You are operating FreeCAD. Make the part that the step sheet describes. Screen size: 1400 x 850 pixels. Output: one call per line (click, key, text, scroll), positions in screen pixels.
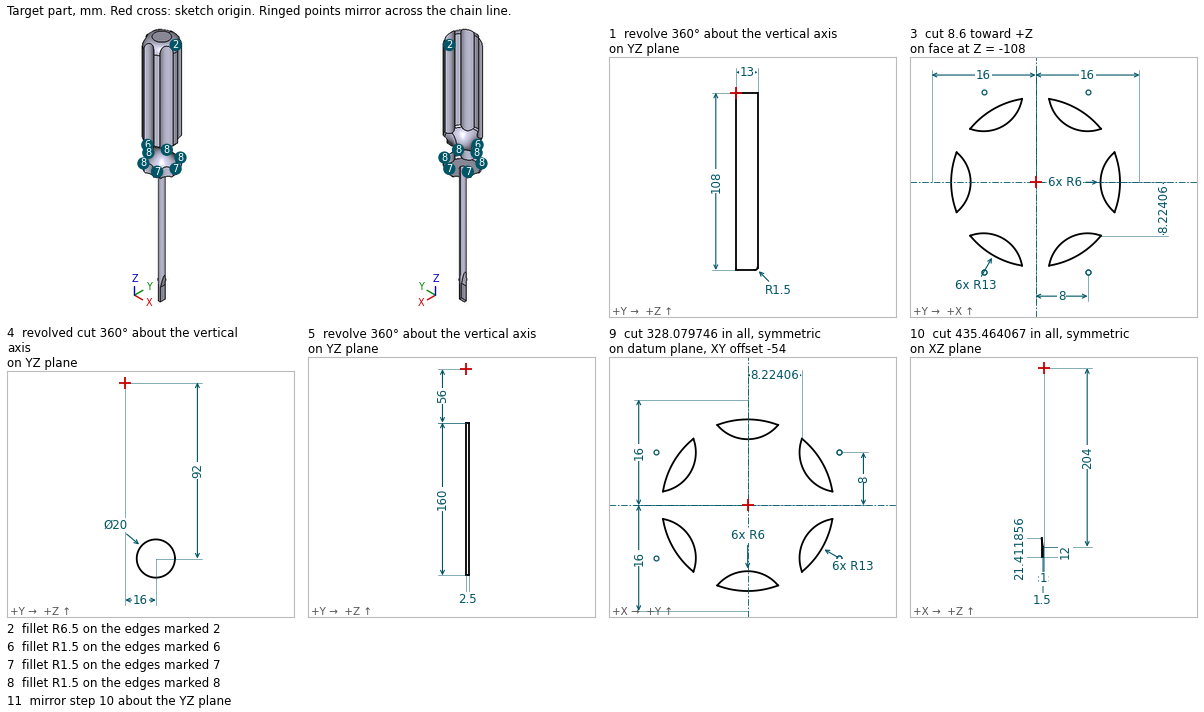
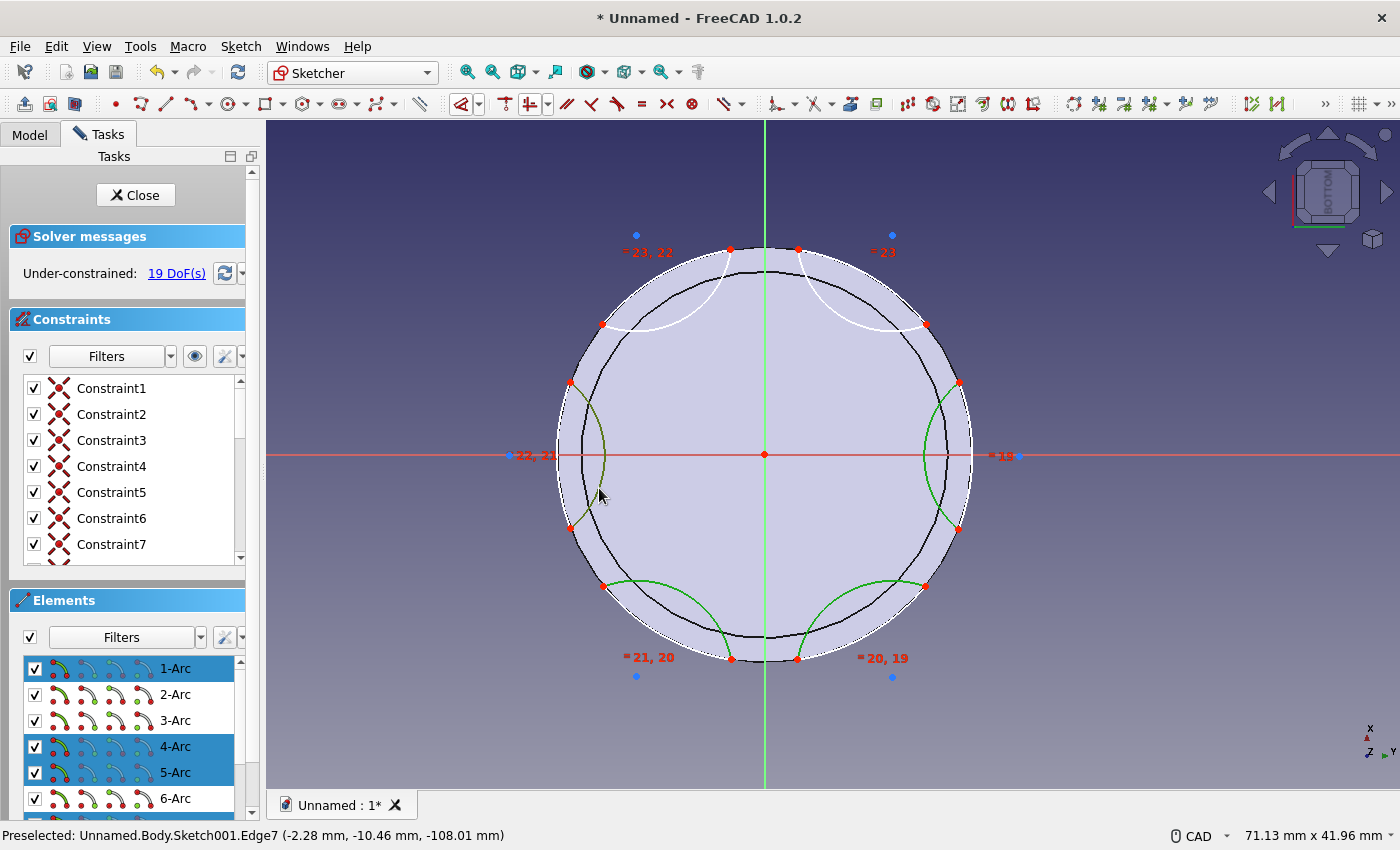
click(653, 330)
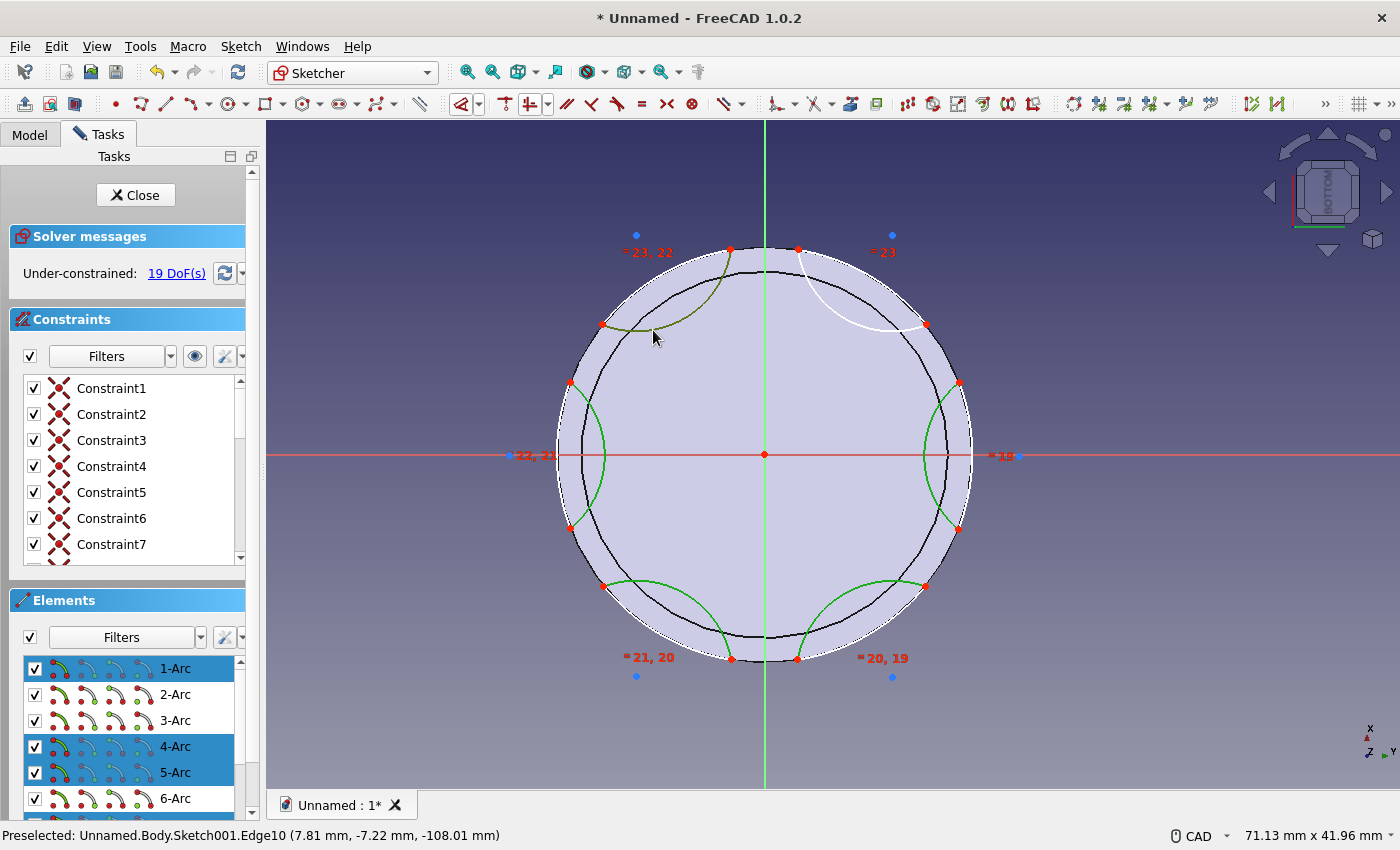
click(818, 296)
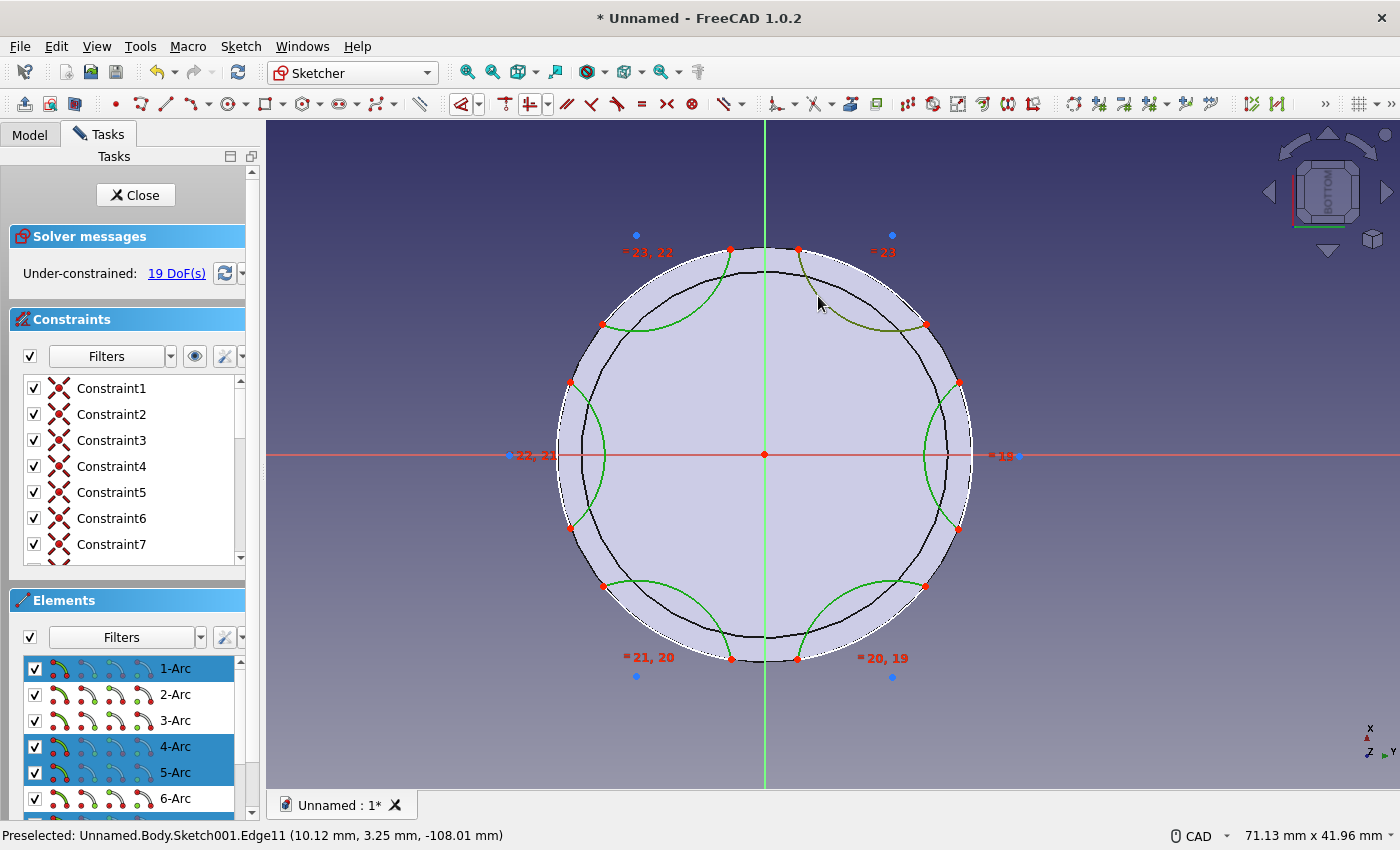
click(642, 104)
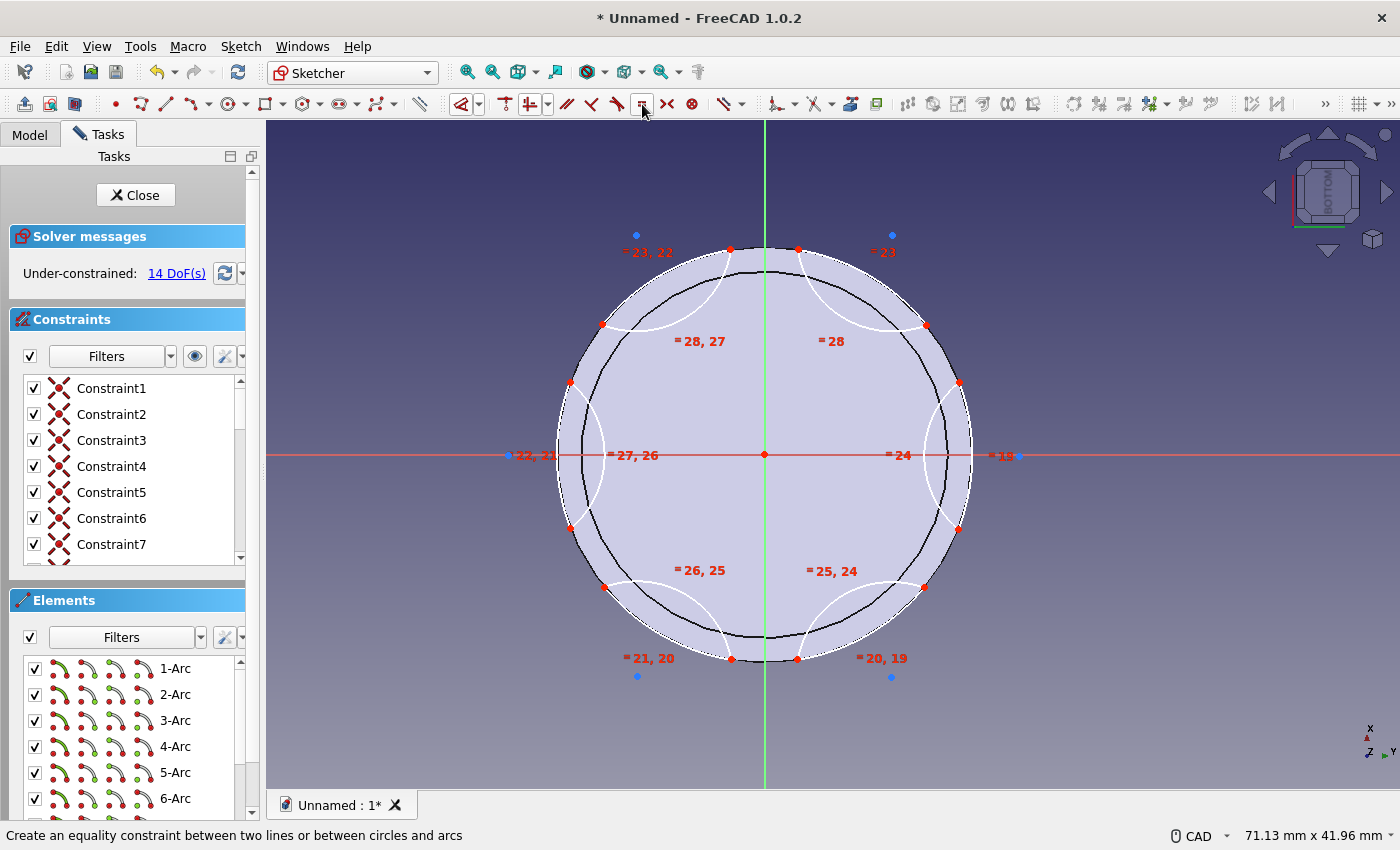
click(1020, 456)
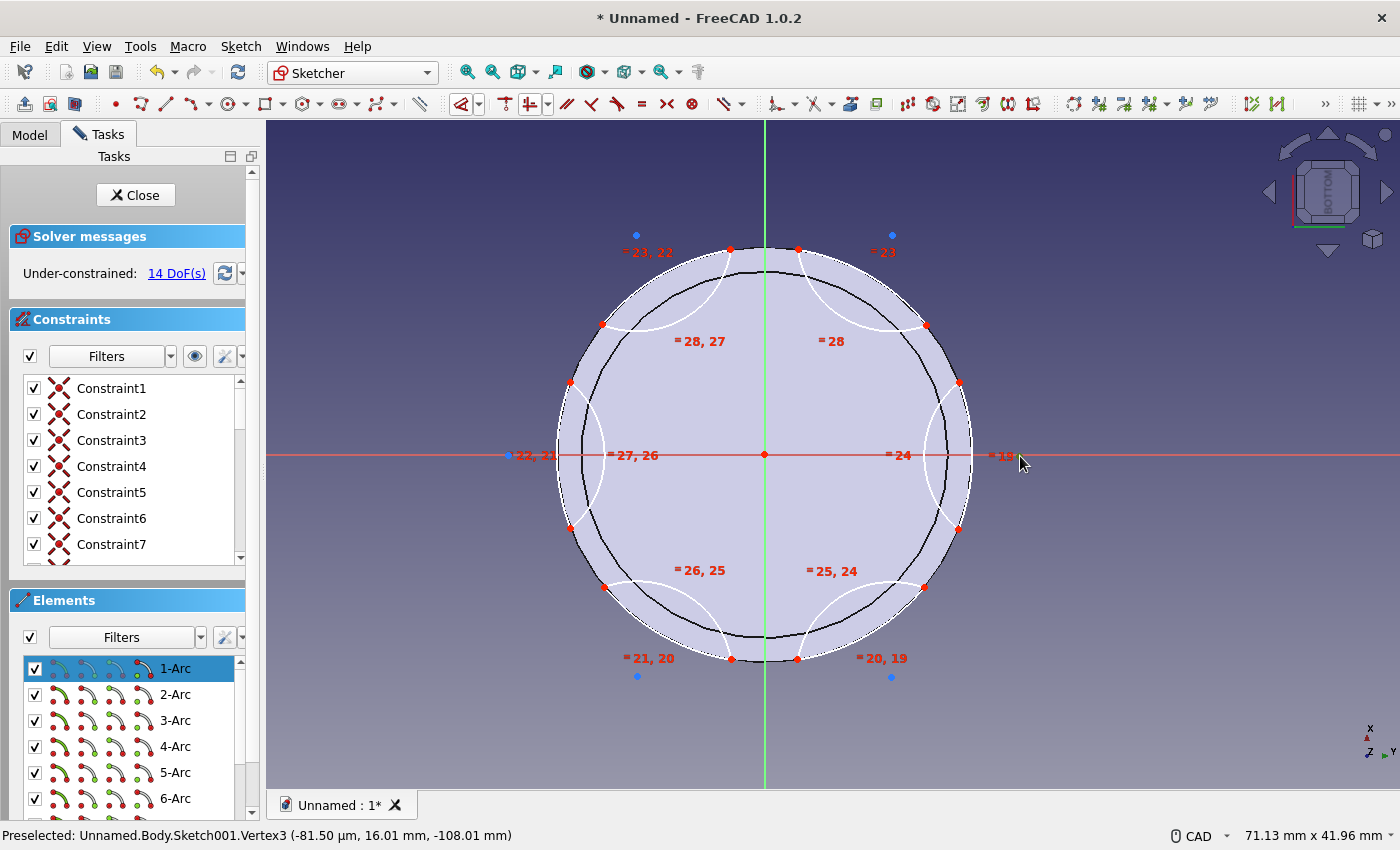
click(361, 455)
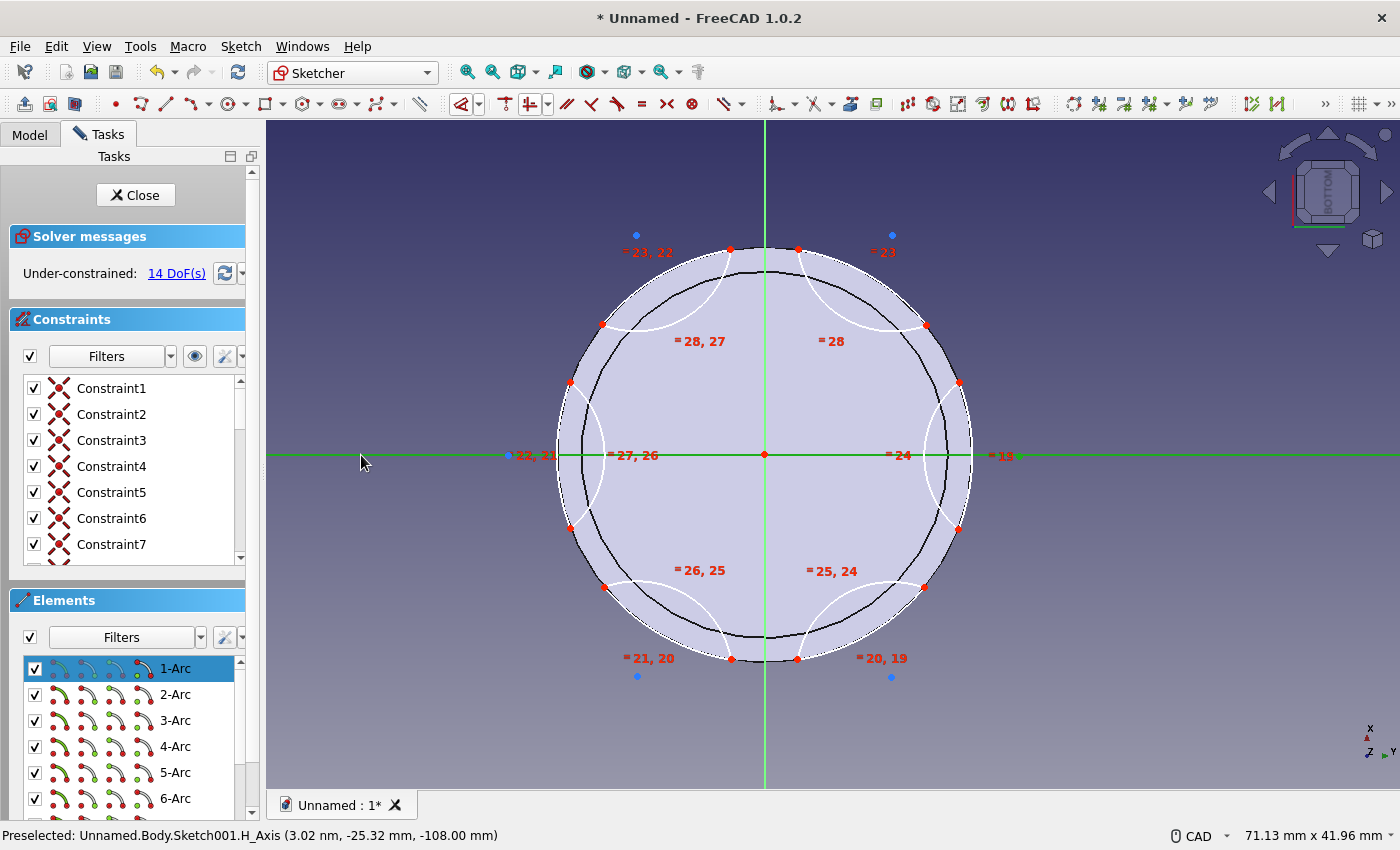
key(c)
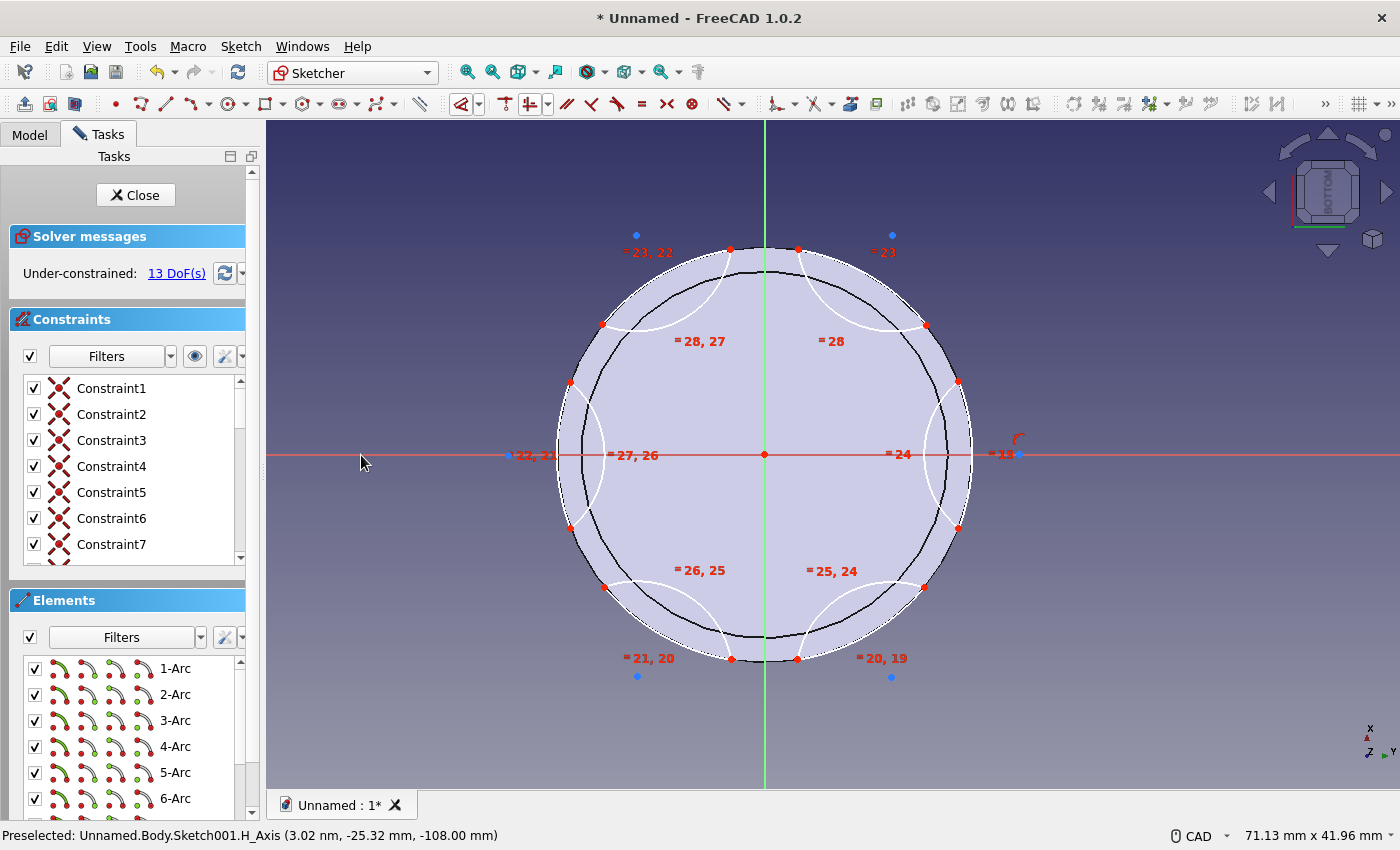
click(509, 456)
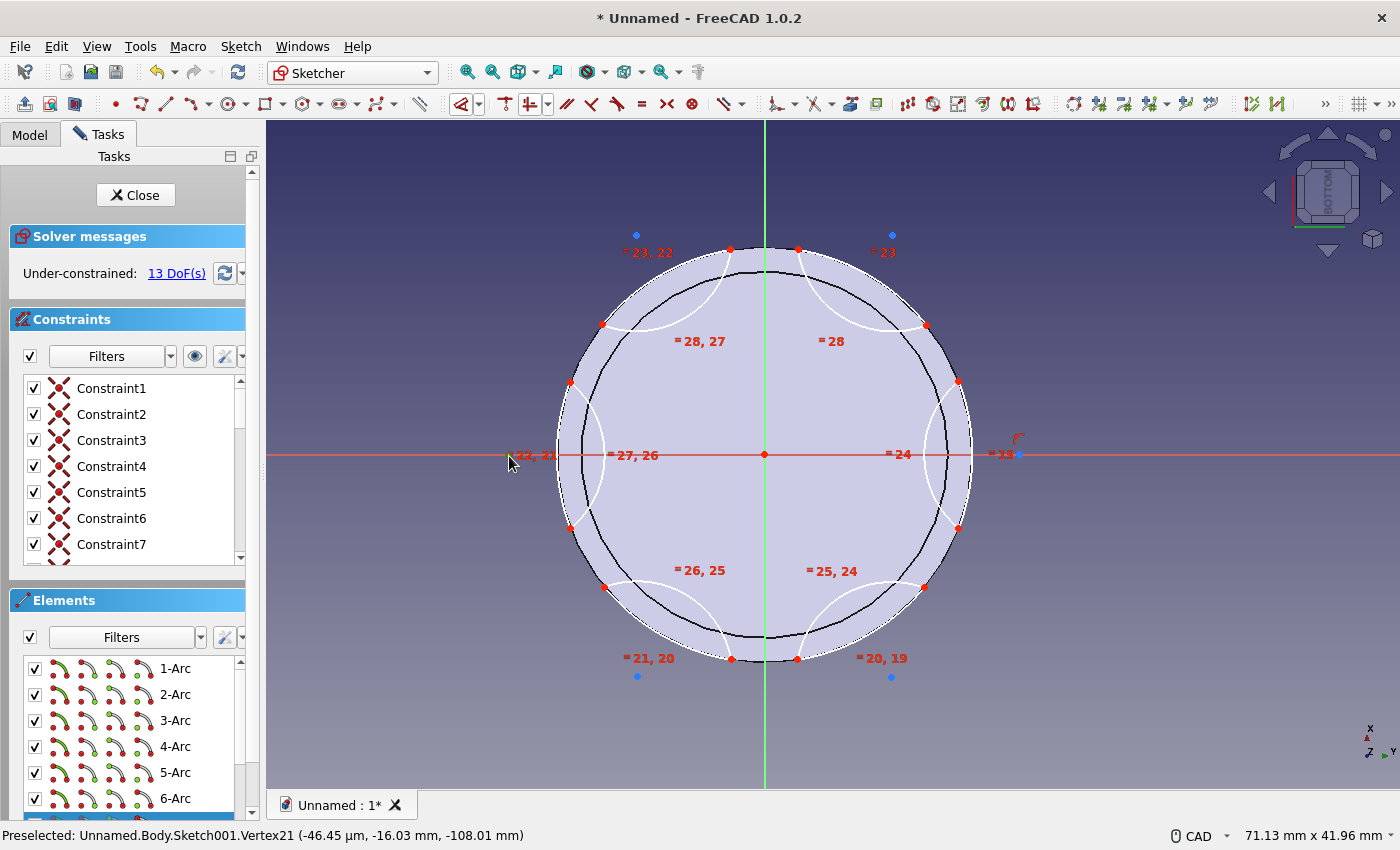
click(361, 455)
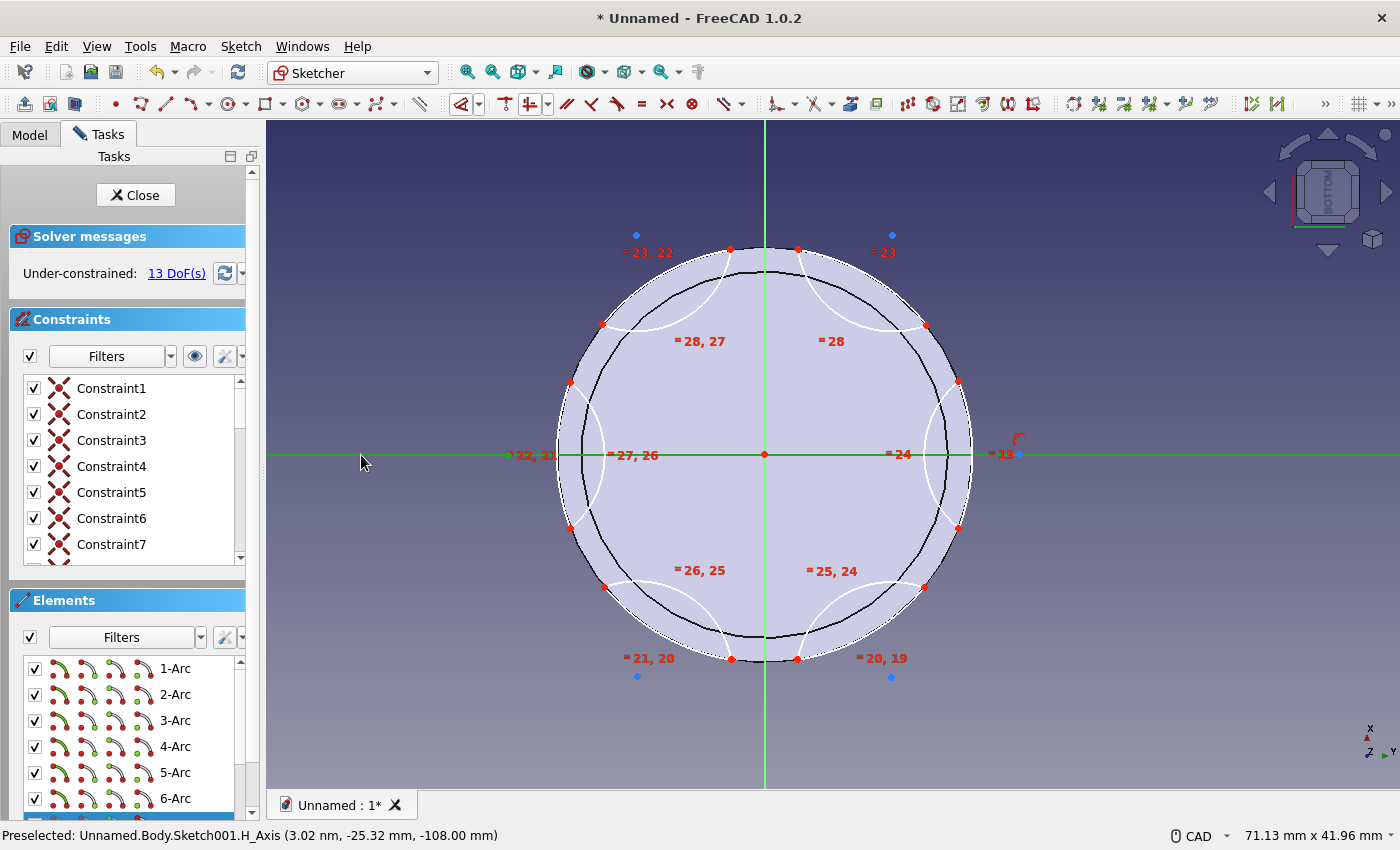
key(c)